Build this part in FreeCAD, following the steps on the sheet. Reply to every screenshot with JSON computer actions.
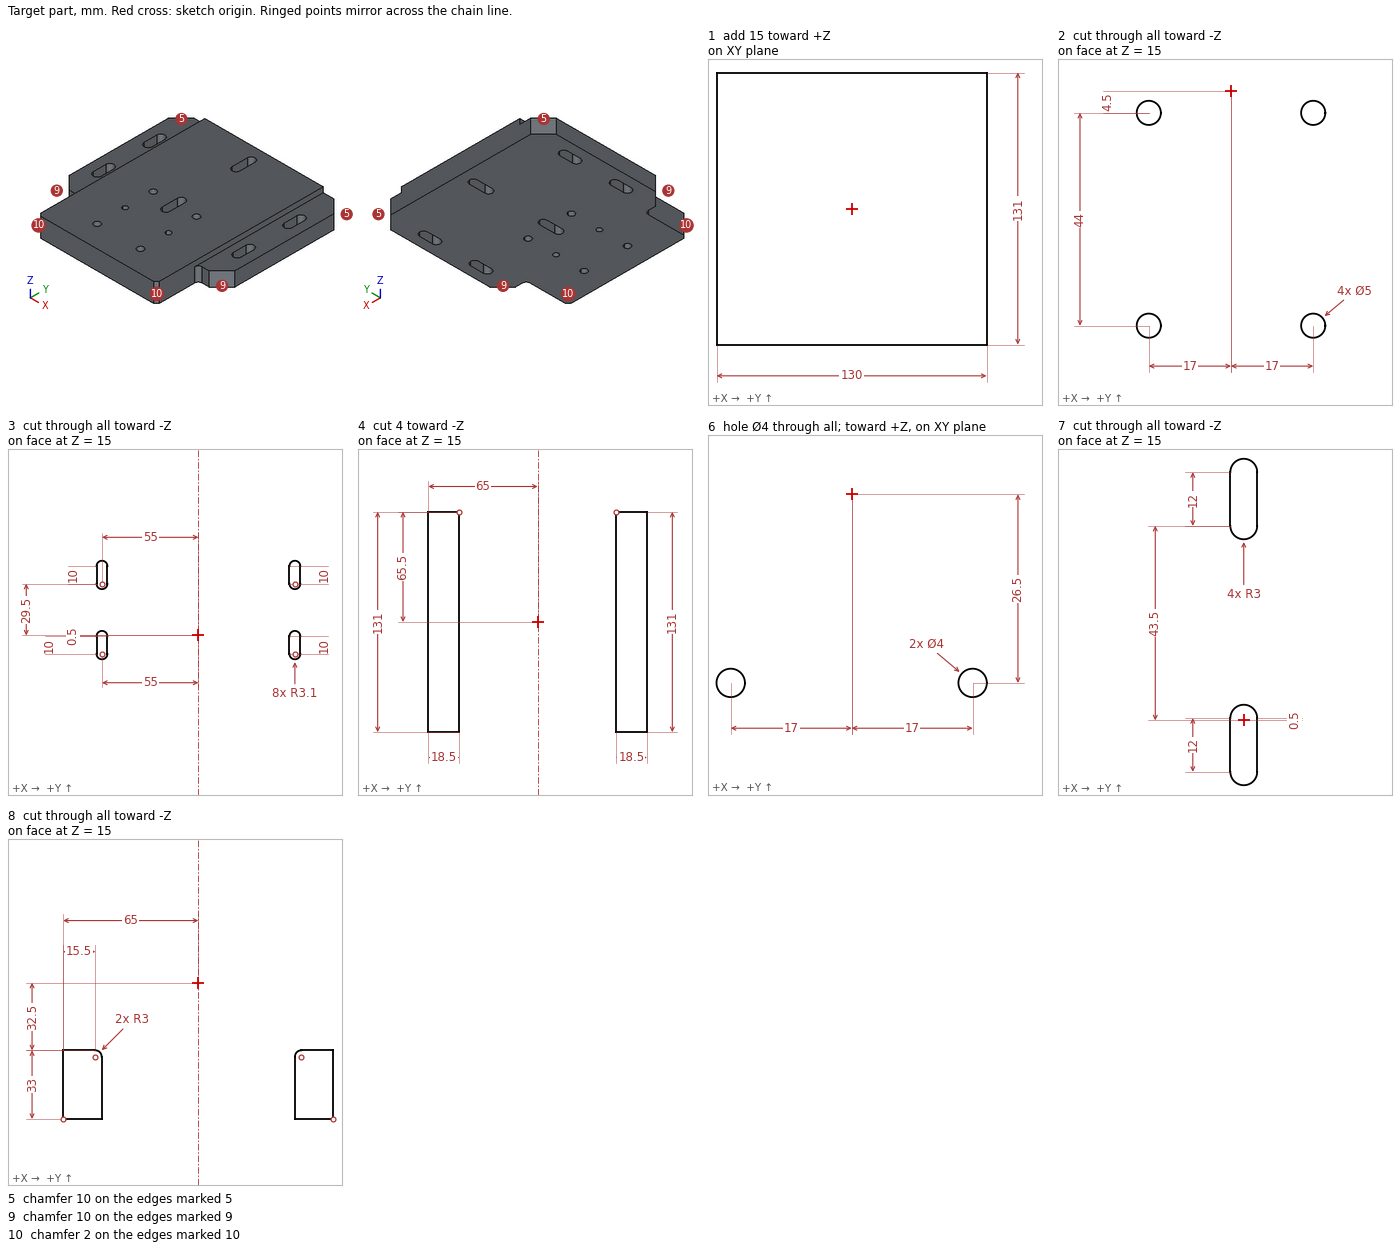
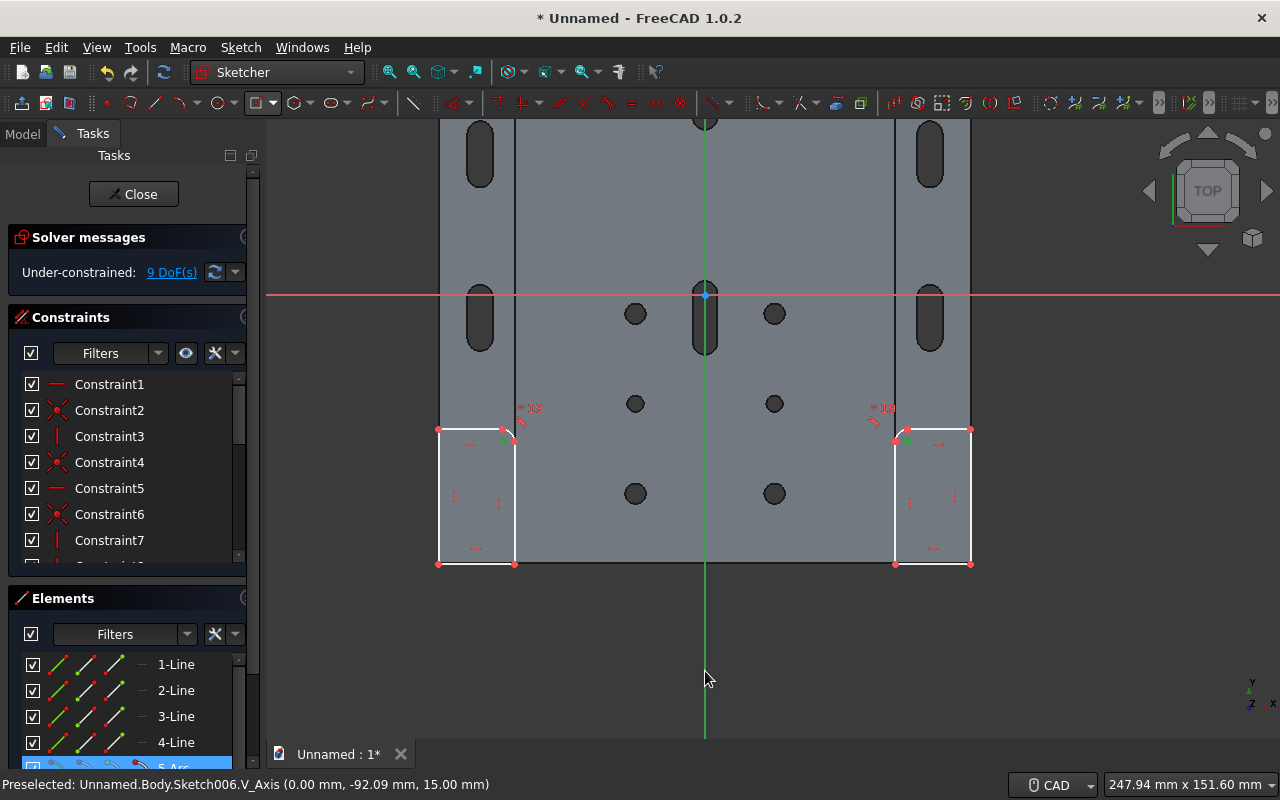
{"action": "left_click", "coordinate": [656, 104]}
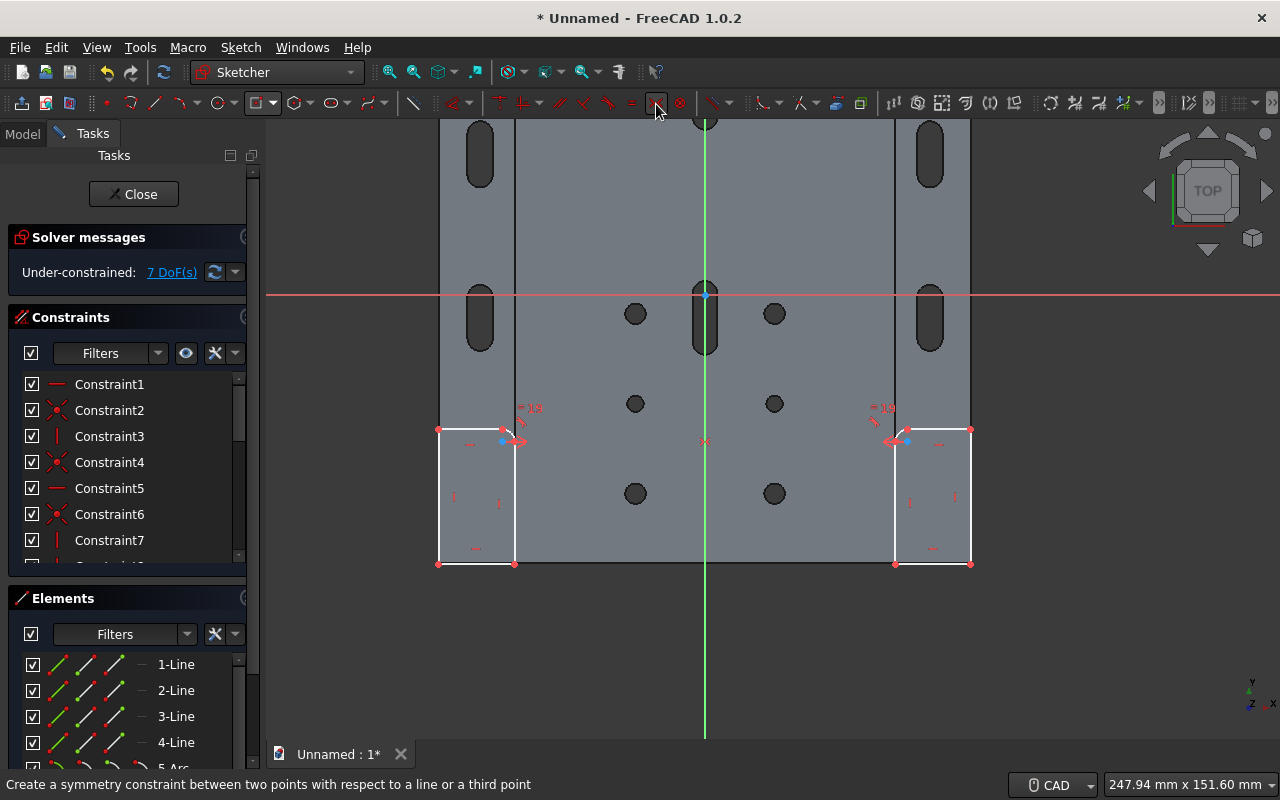
{"action": "left_click", "coordinate": [439, 564]}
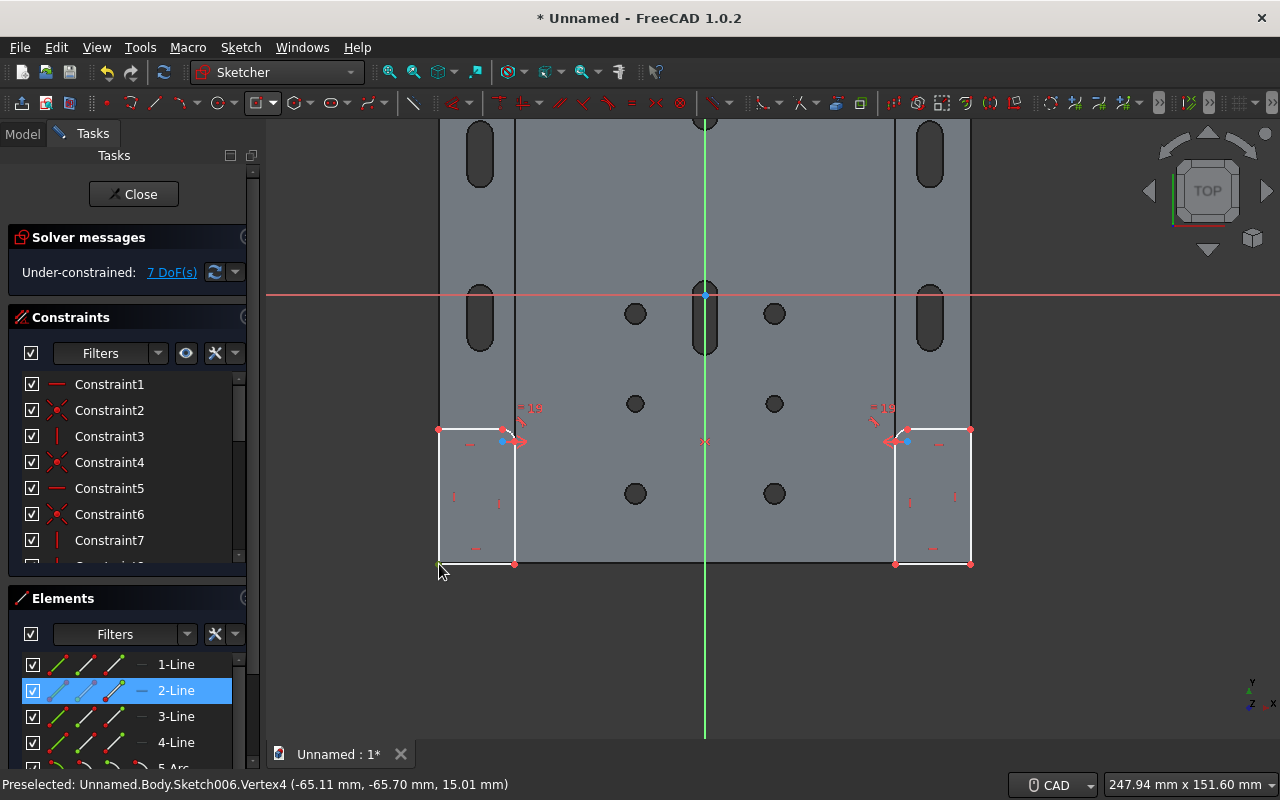
{"action": "left_click", "coordinate": [971, 564]}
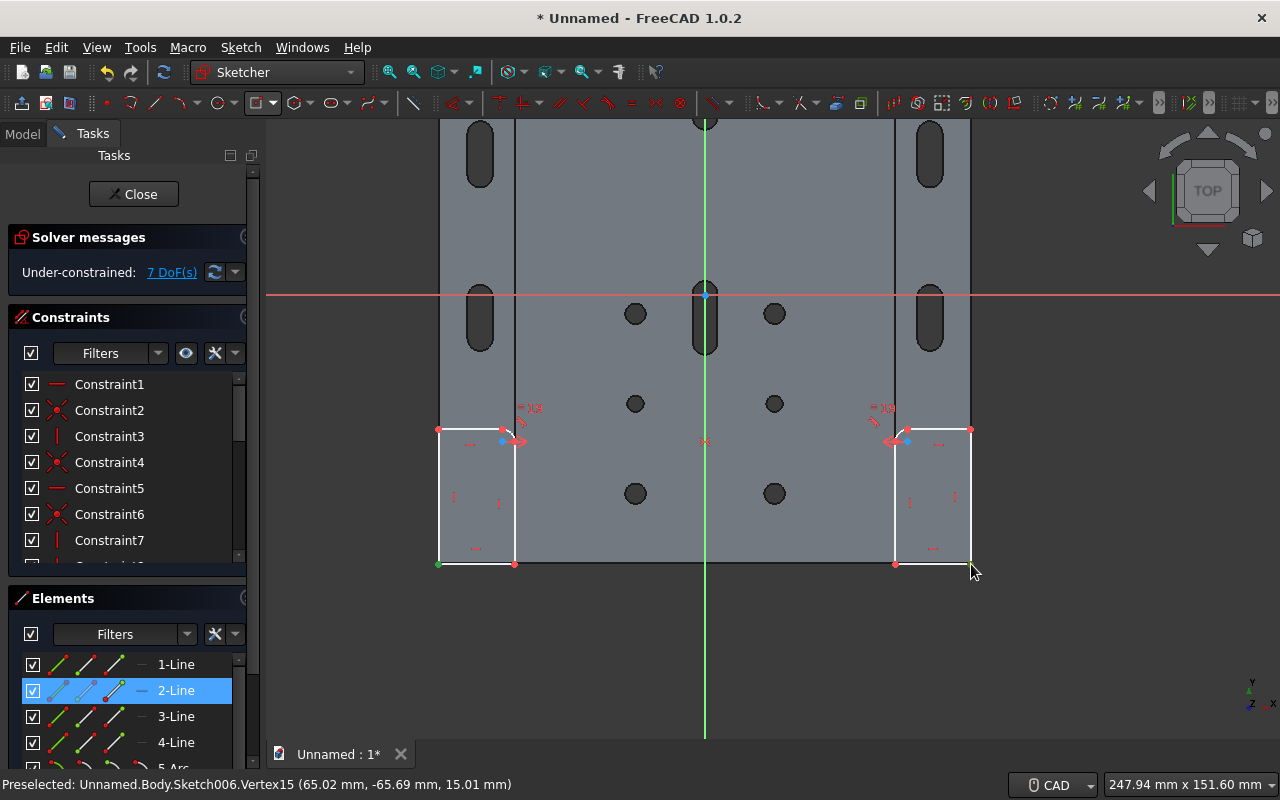
{"action": "left_click", "coordinate": [705, 671]}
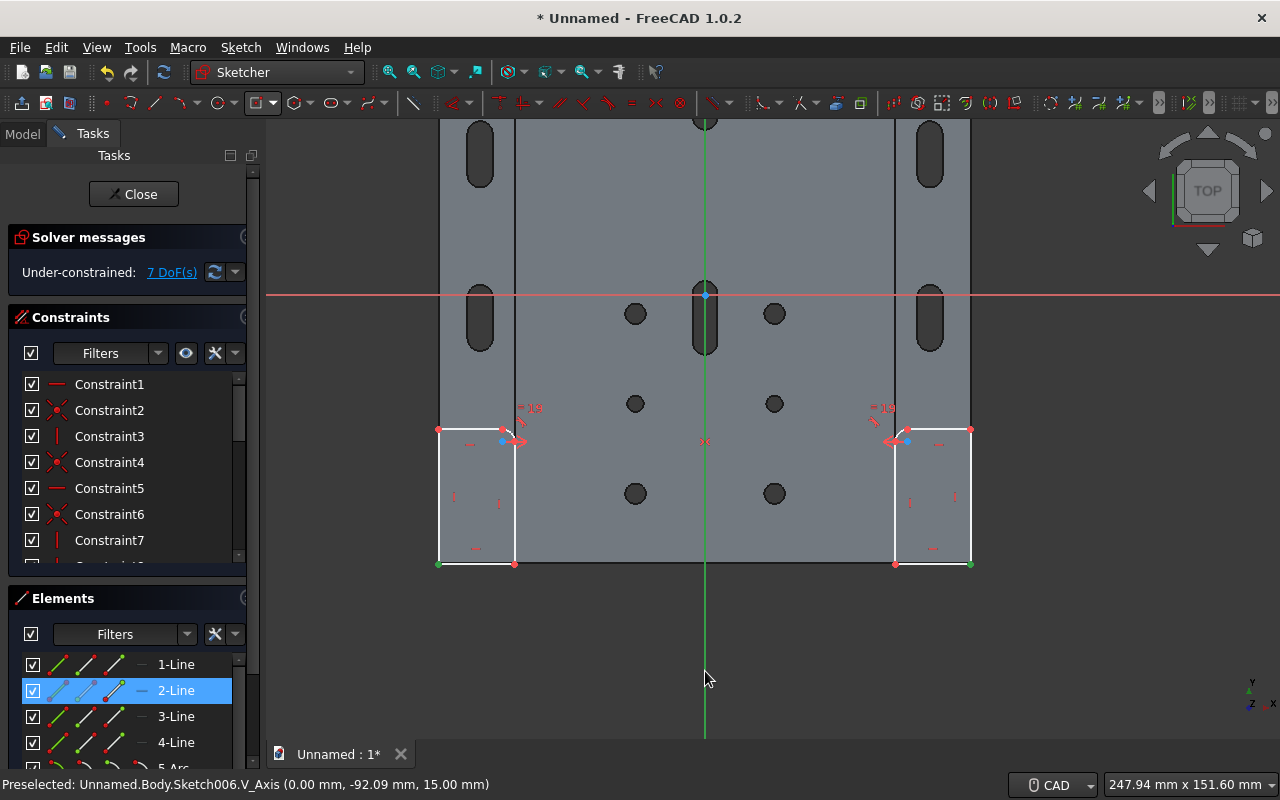
{"action": "key", "text": "s"}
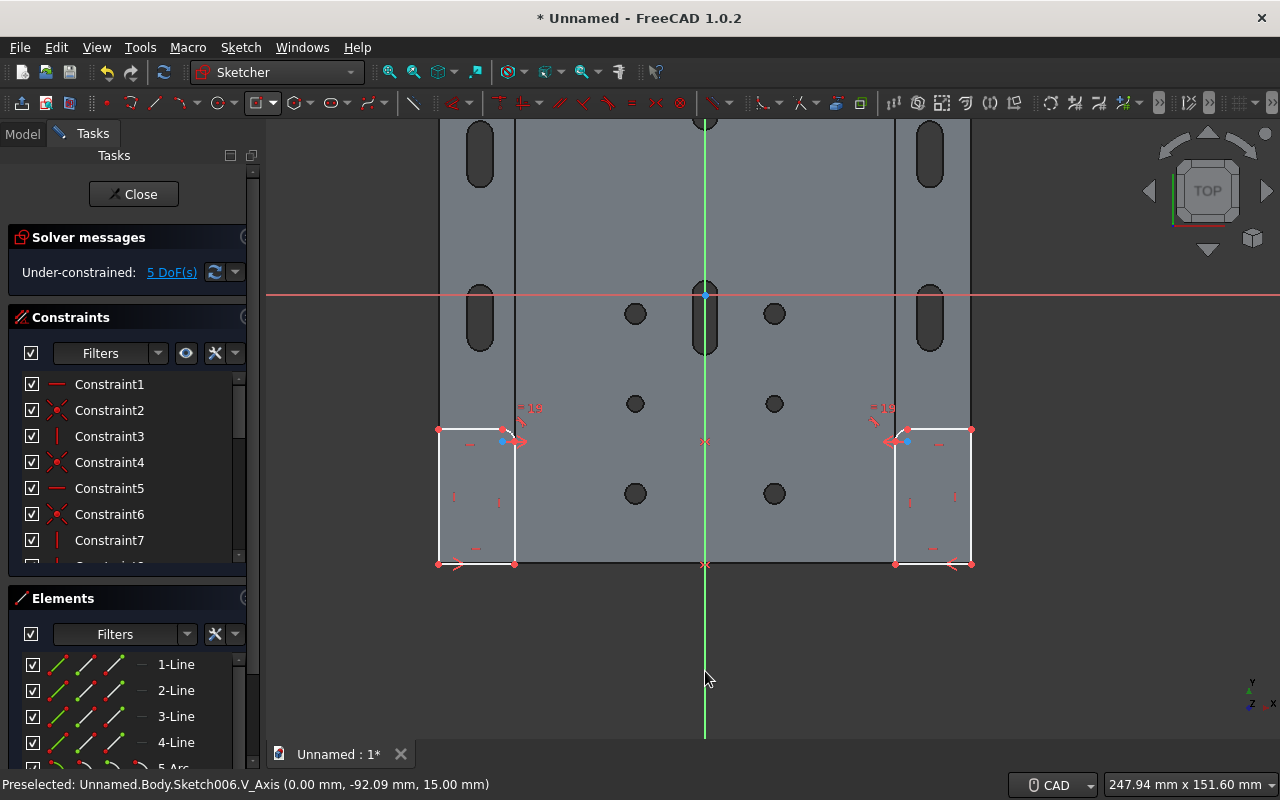
{"action": "left_click", "coordinate": [452, 104]}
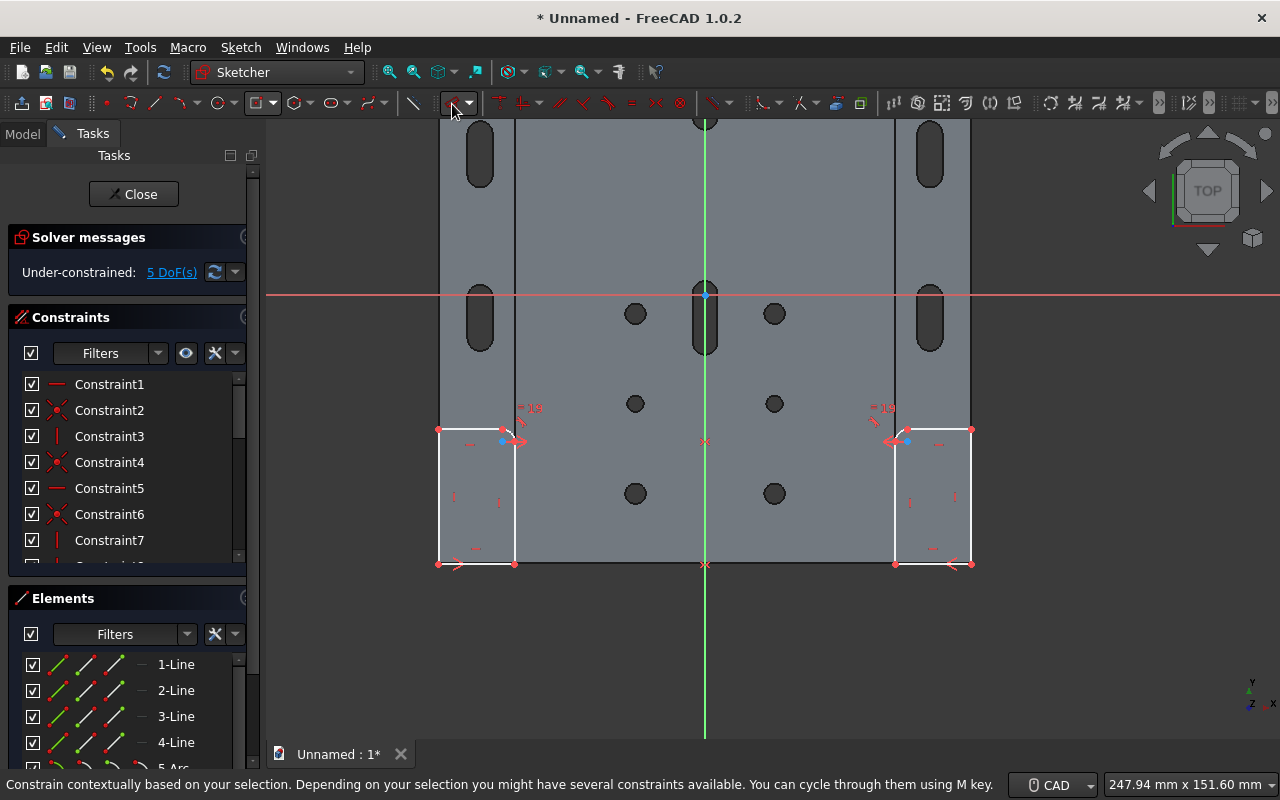
{"action": "scroll", "coordinate": [511, 433], "scroll_direction": "up", "scroll_amount": 6}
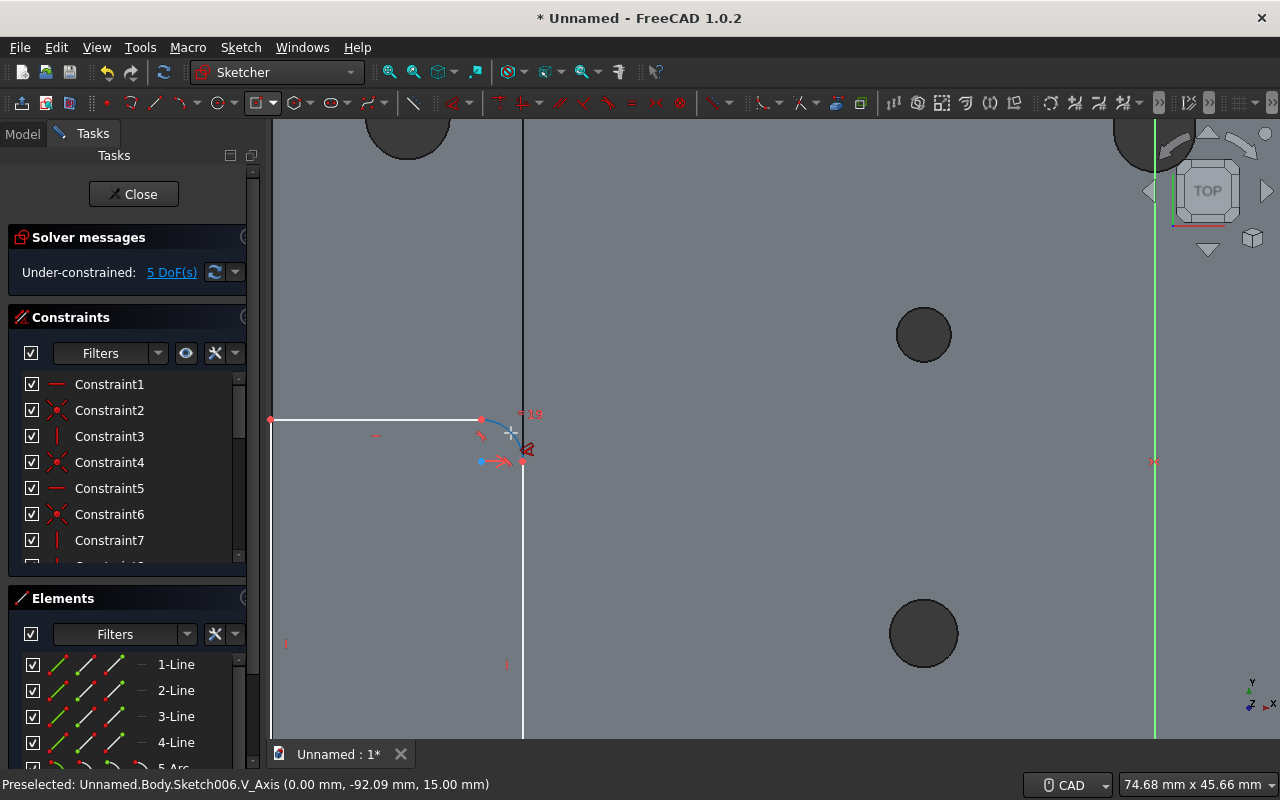
{"action": "left_click", "coordinate": [511, 432]}
{"action": "left_click", "coordinate": [534, 409]}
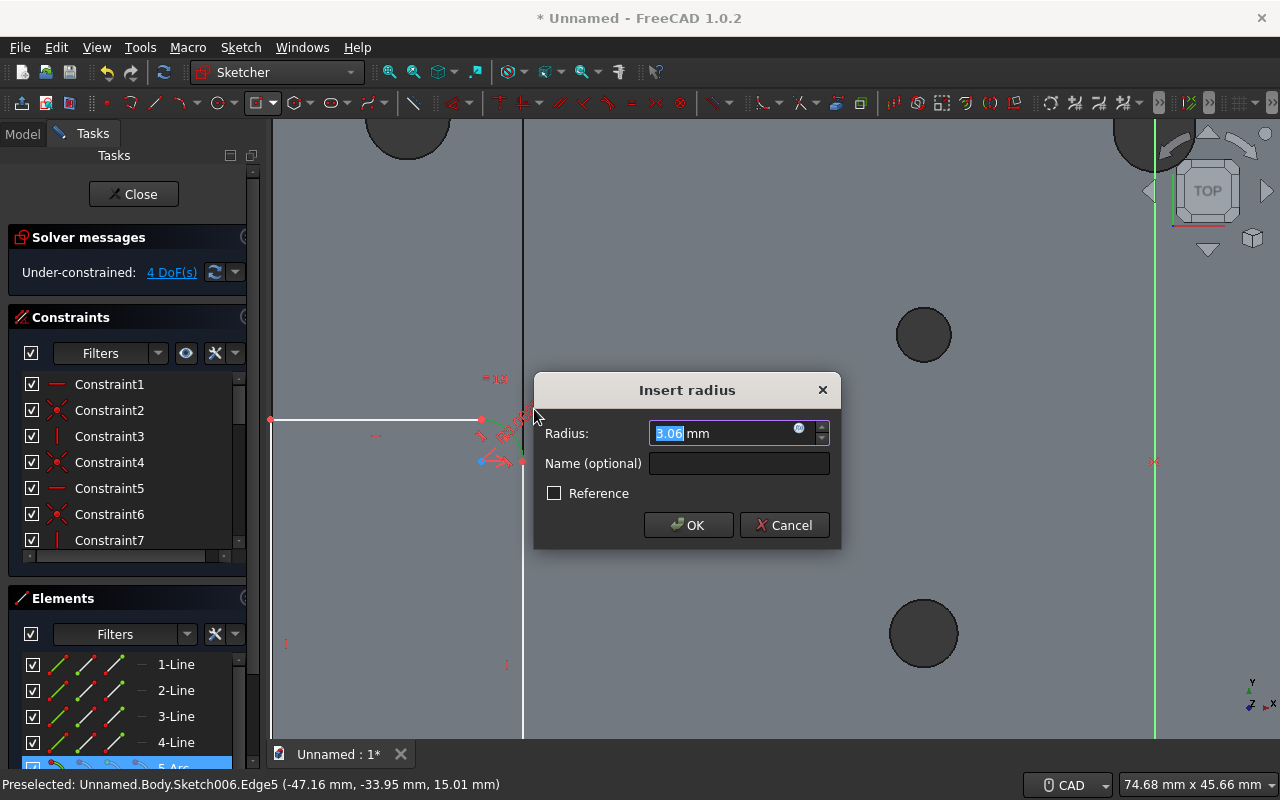
{"action": "type", "text": "3"}
{"action": "key", "text": "Return"}